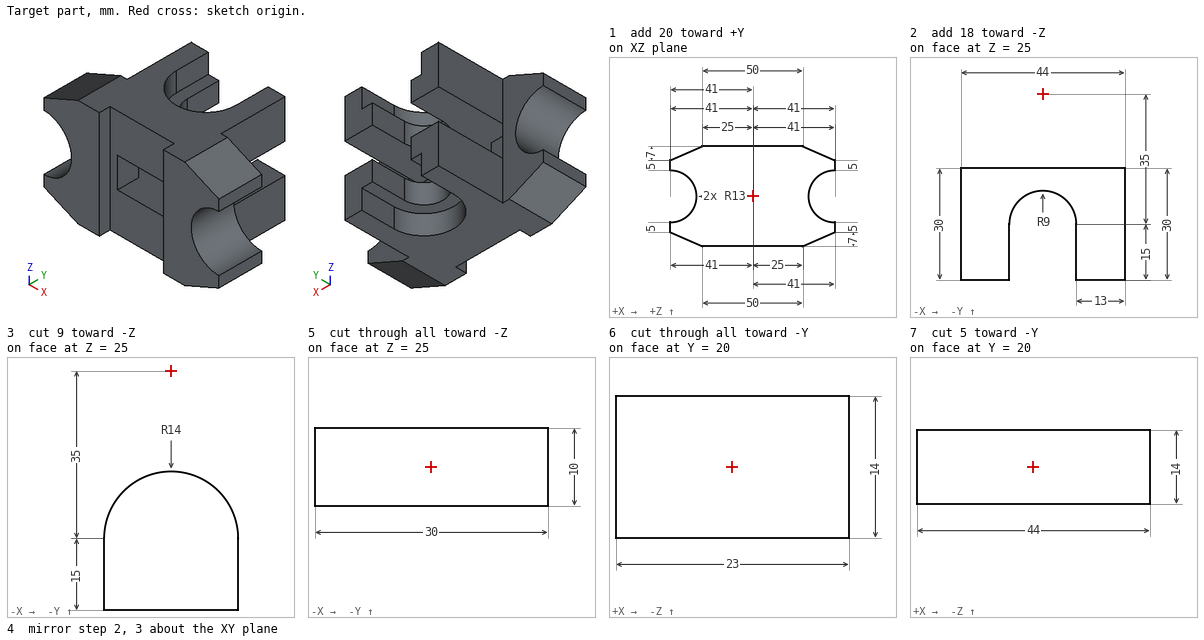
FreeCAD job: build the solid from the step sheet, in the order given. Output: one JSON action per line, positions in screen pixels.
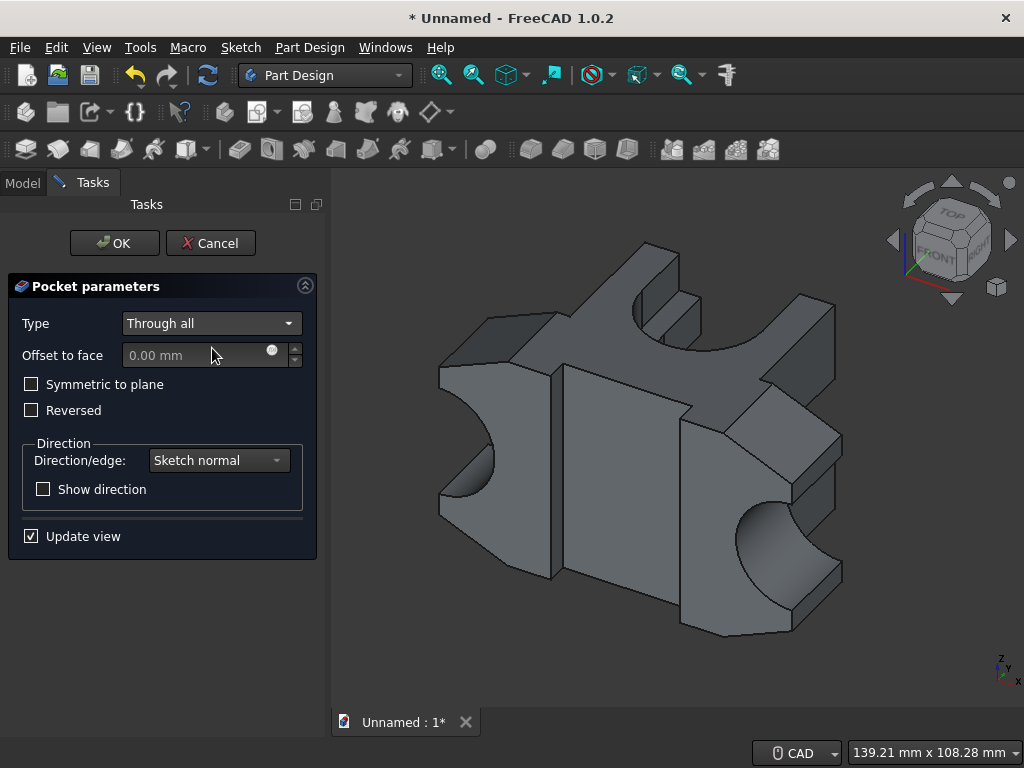
{"action": "left_click", "coordinate": [115, 243]}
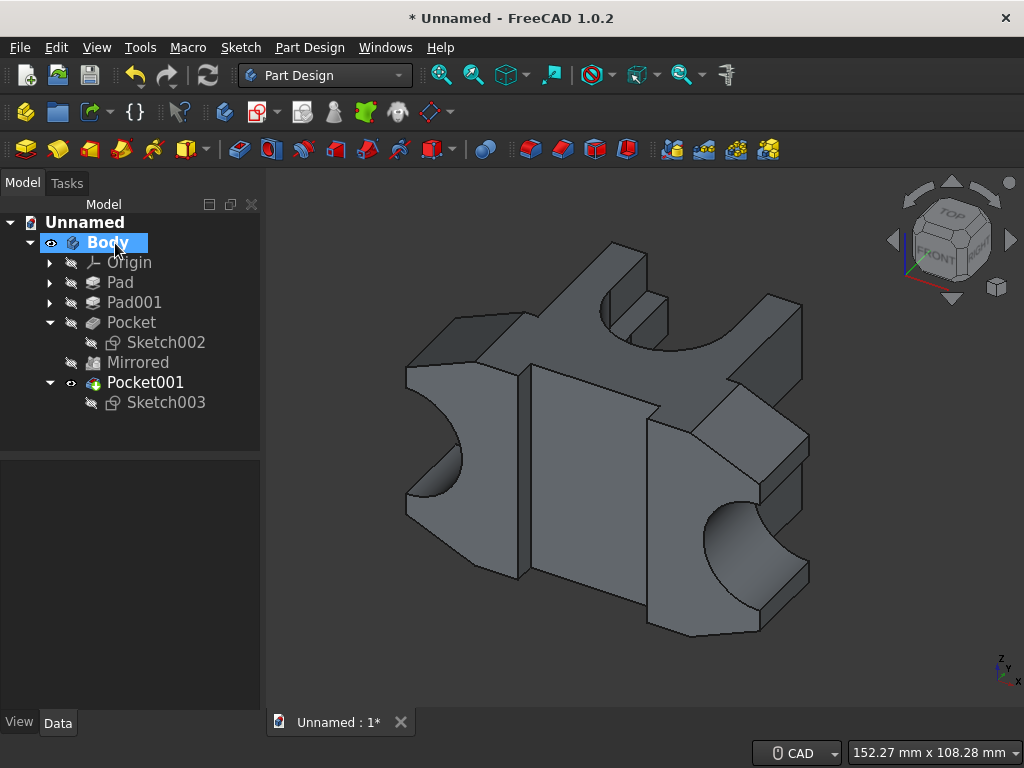
{"action": "key", "text": "4"}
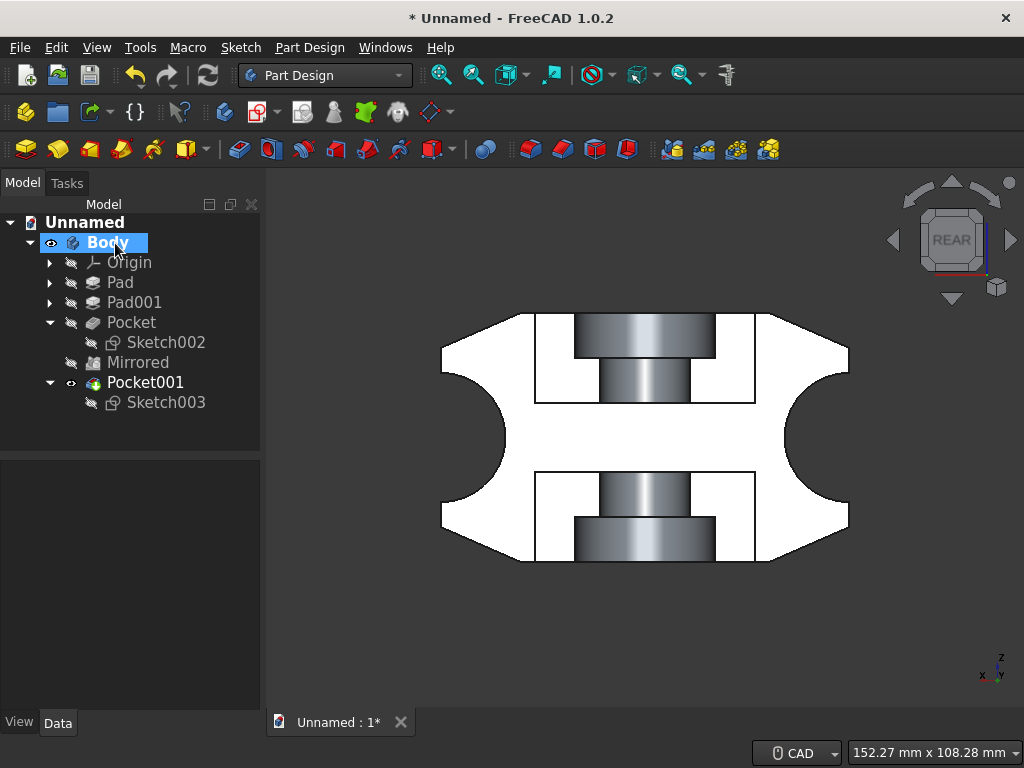
{"action": "left_click", "coordinate": [587, 437]}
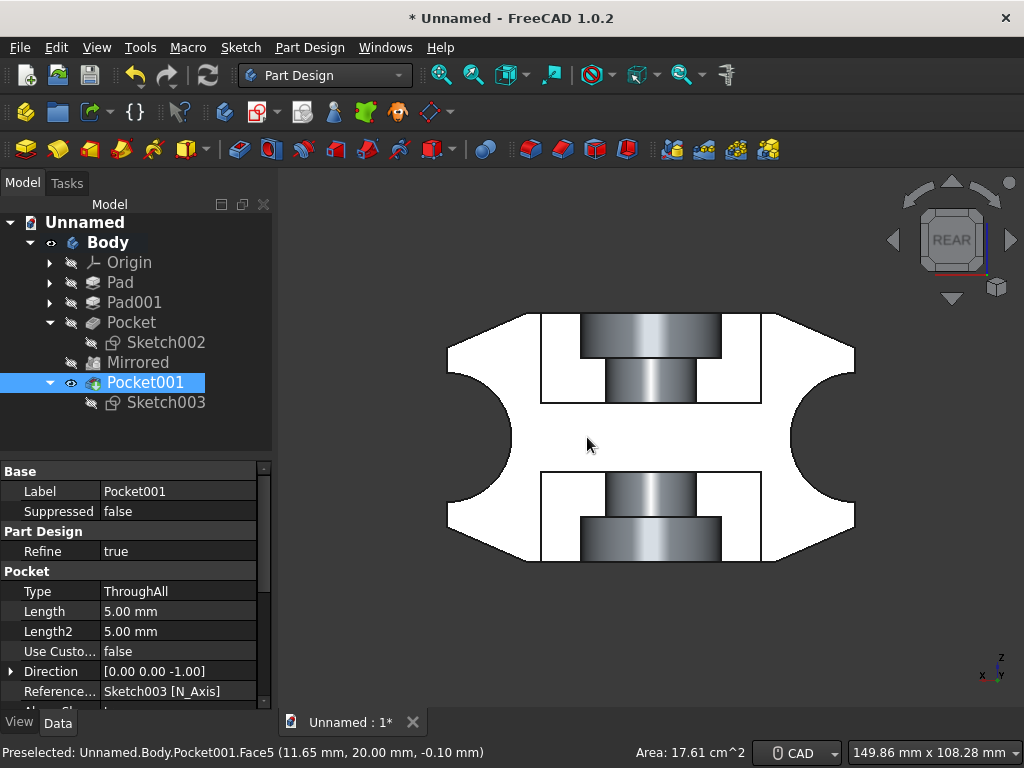
{"action": "left_click", "coordinate": [258, 112]}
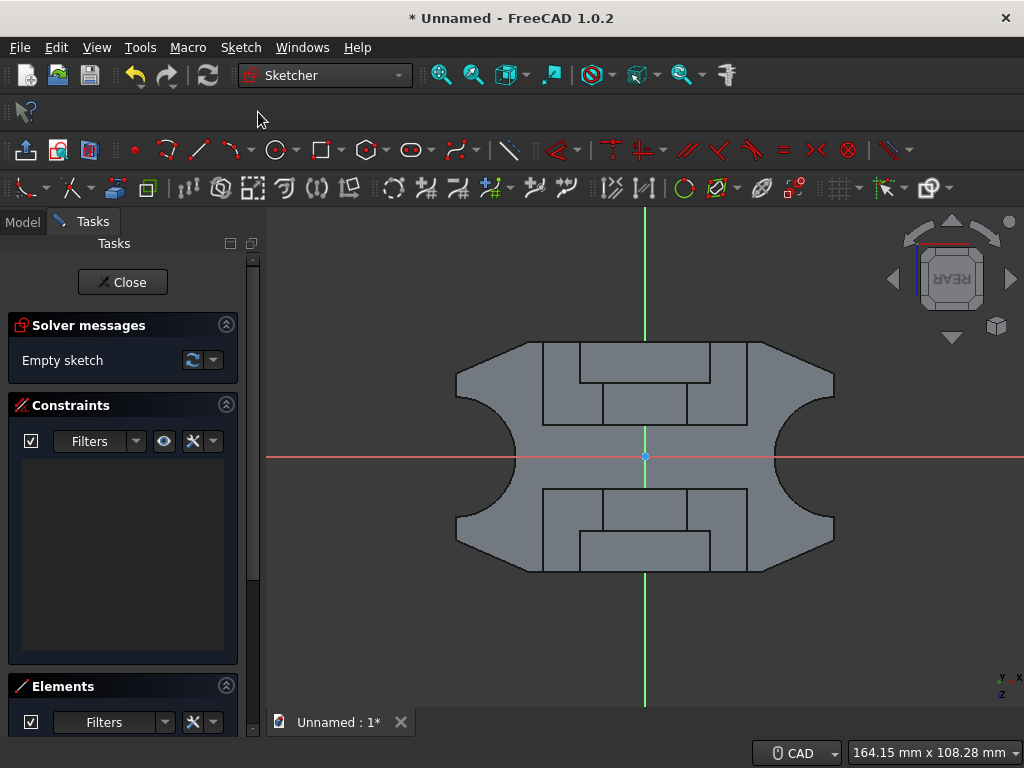
{"action": "scroll", "coordinate": [667, 457], "scroll_direction": "up", "scroll_amount": 7}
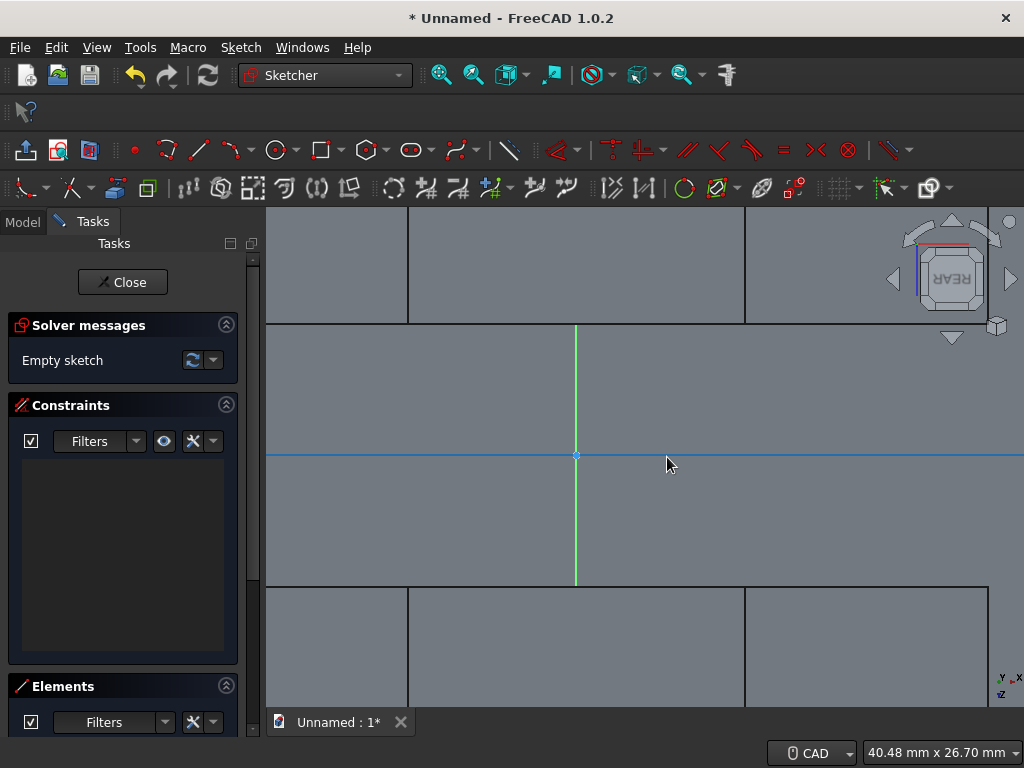
{"action": "key", "text": "g v"}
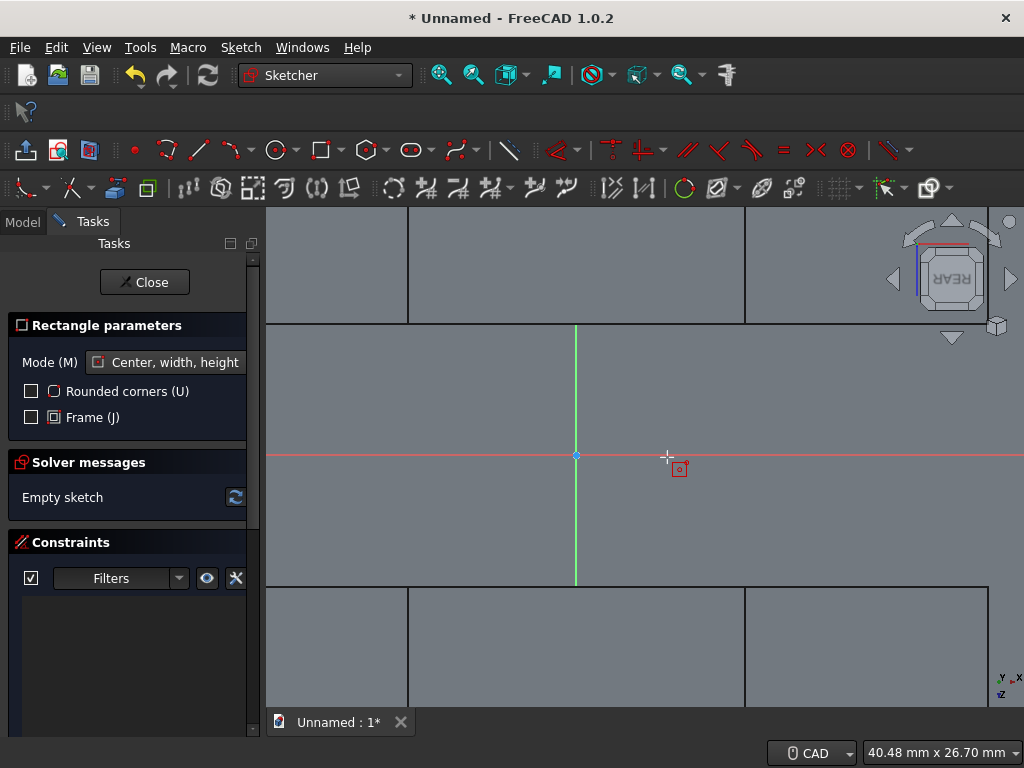
{"action": "left_click", "coordinate": [576, 455]}
{"action": "mouse_move", "coordinate": [792, 324]}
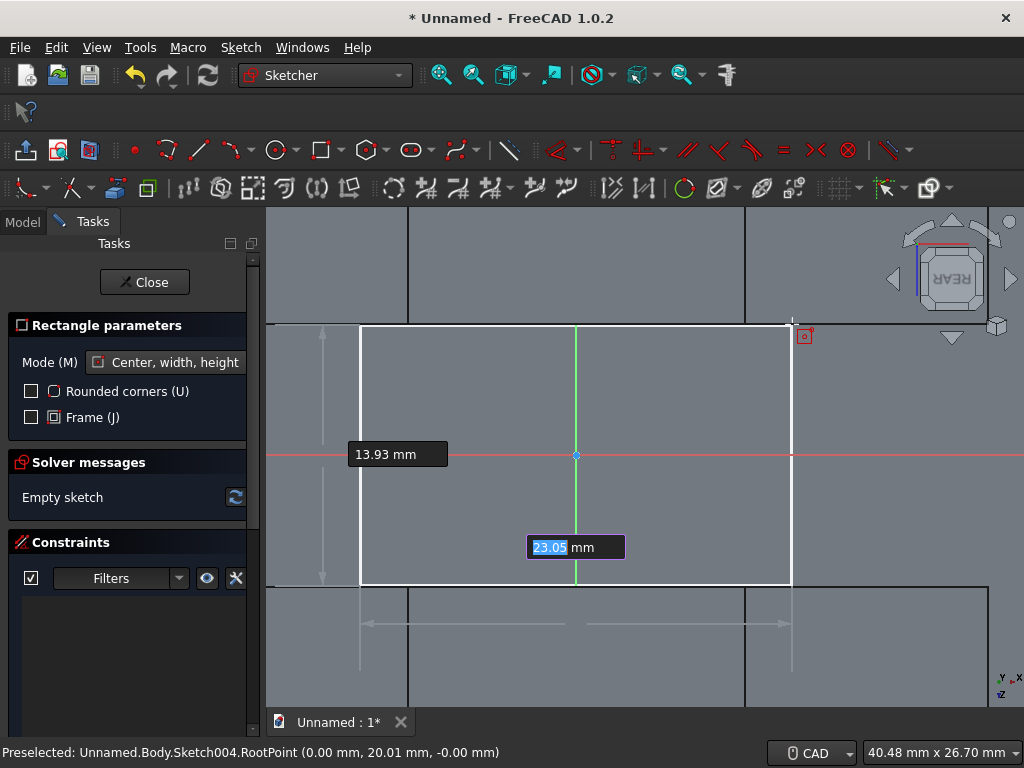
{"action": "type", "text": "23"}
{"action": "key", "text": "Tab"}
{"action": "type", "text": "14"}
{"action": "key", "text": "Return"}
{"action": "key", "text": "Escape"}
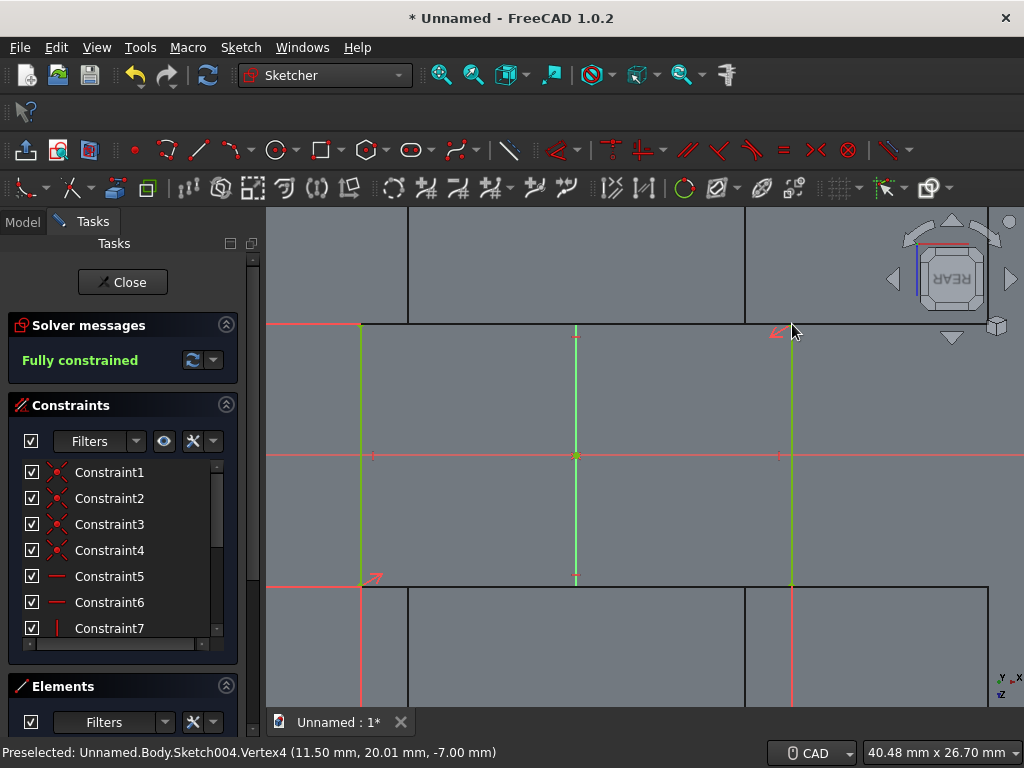
{"action": "left_click", "coordinate": [123, 282]}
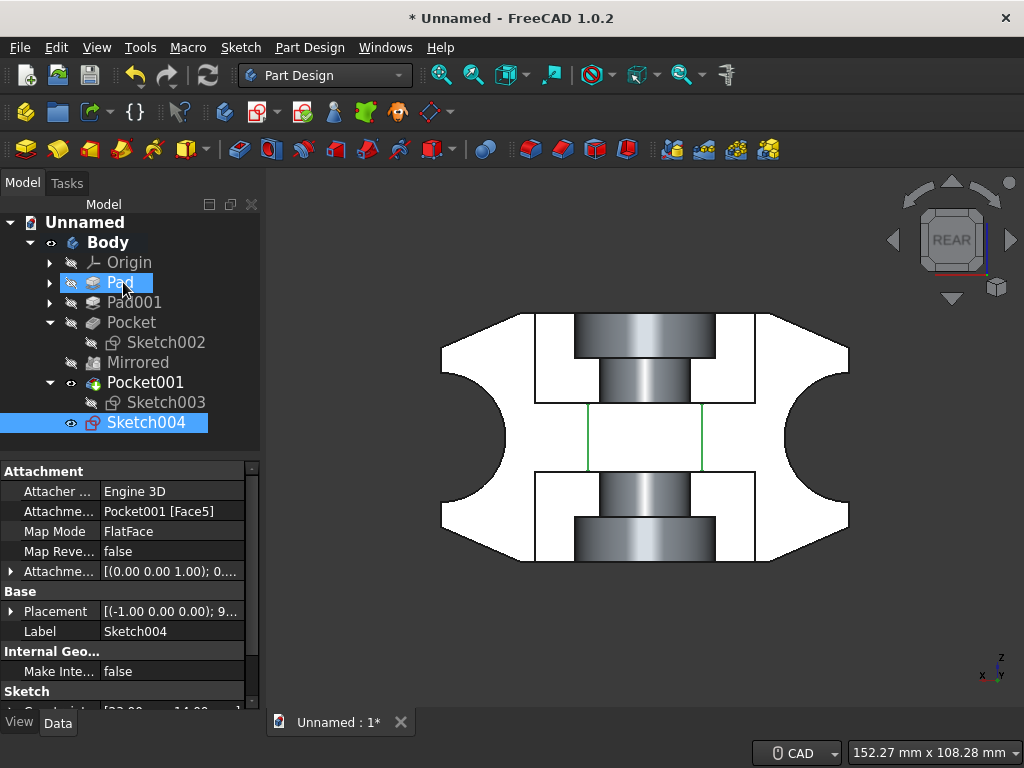
{"action": "left_click", "coordinate": [240, 150]}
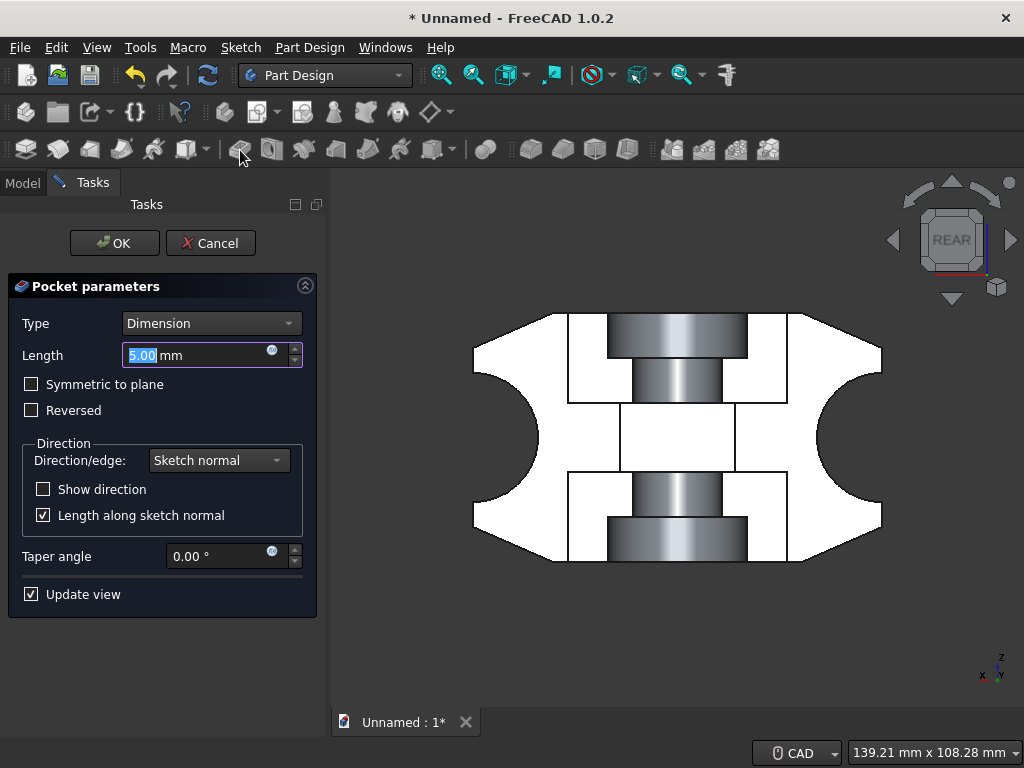
{"action": "left_click", "coordinate": [212, 324]}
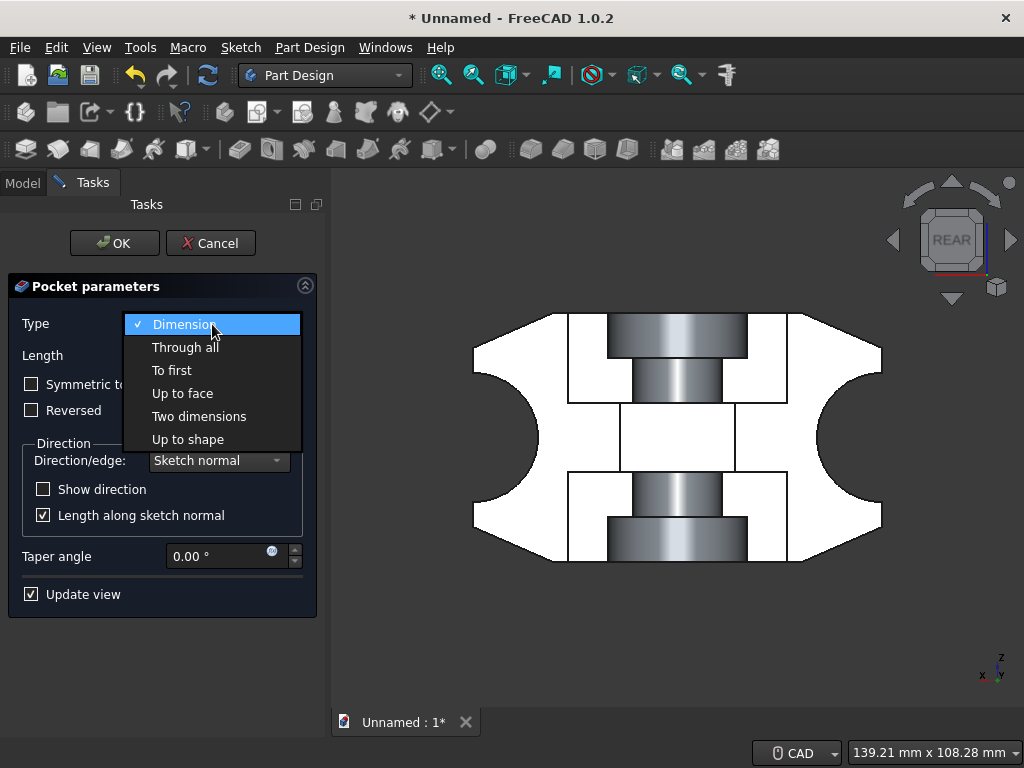
{"action": "left_click", "coordinate": [212, 348]}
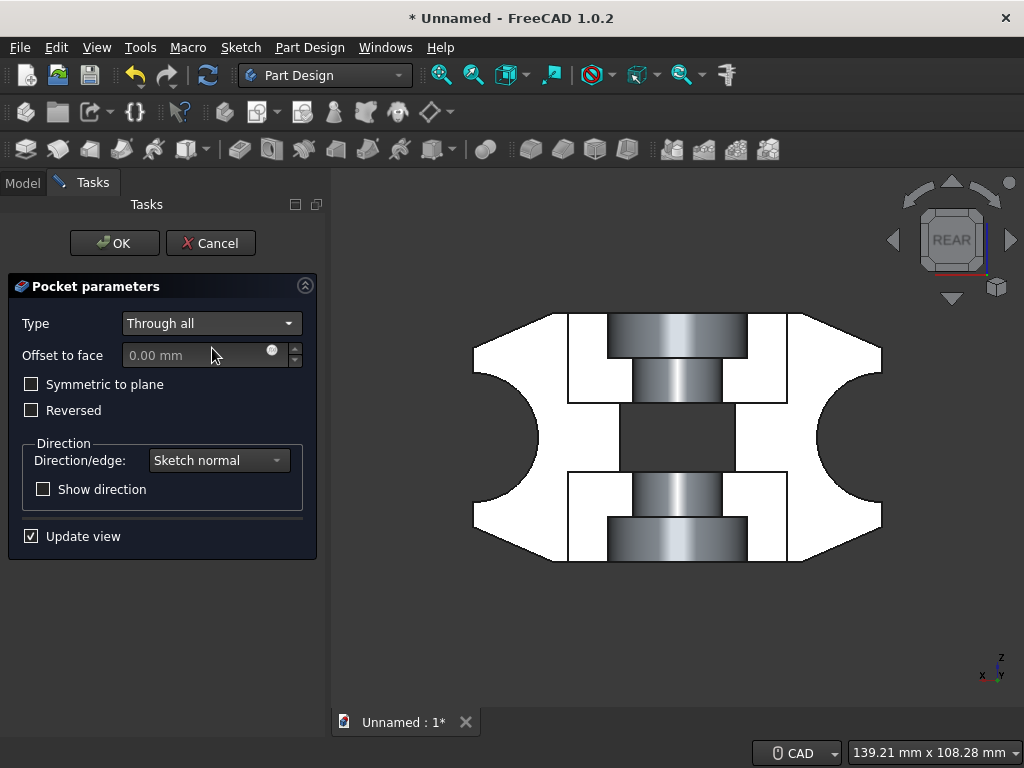
{"action": "left_click", "coordinate": [115, 243]}